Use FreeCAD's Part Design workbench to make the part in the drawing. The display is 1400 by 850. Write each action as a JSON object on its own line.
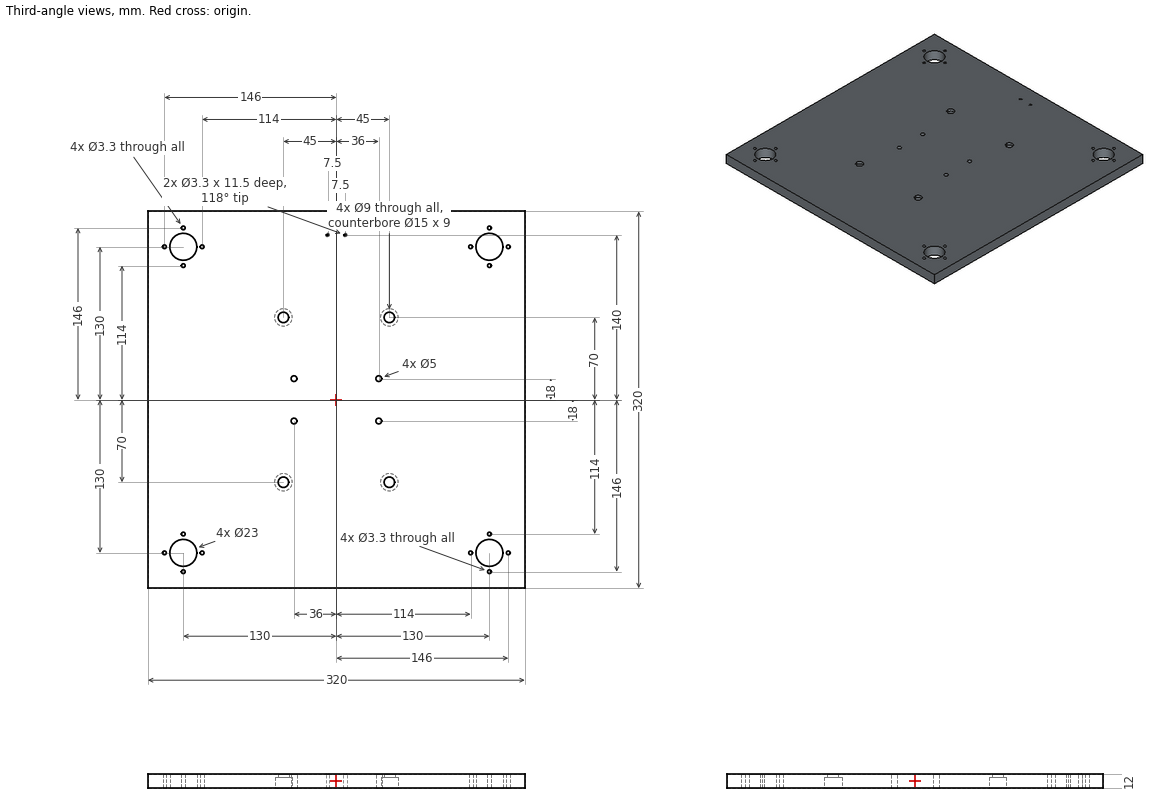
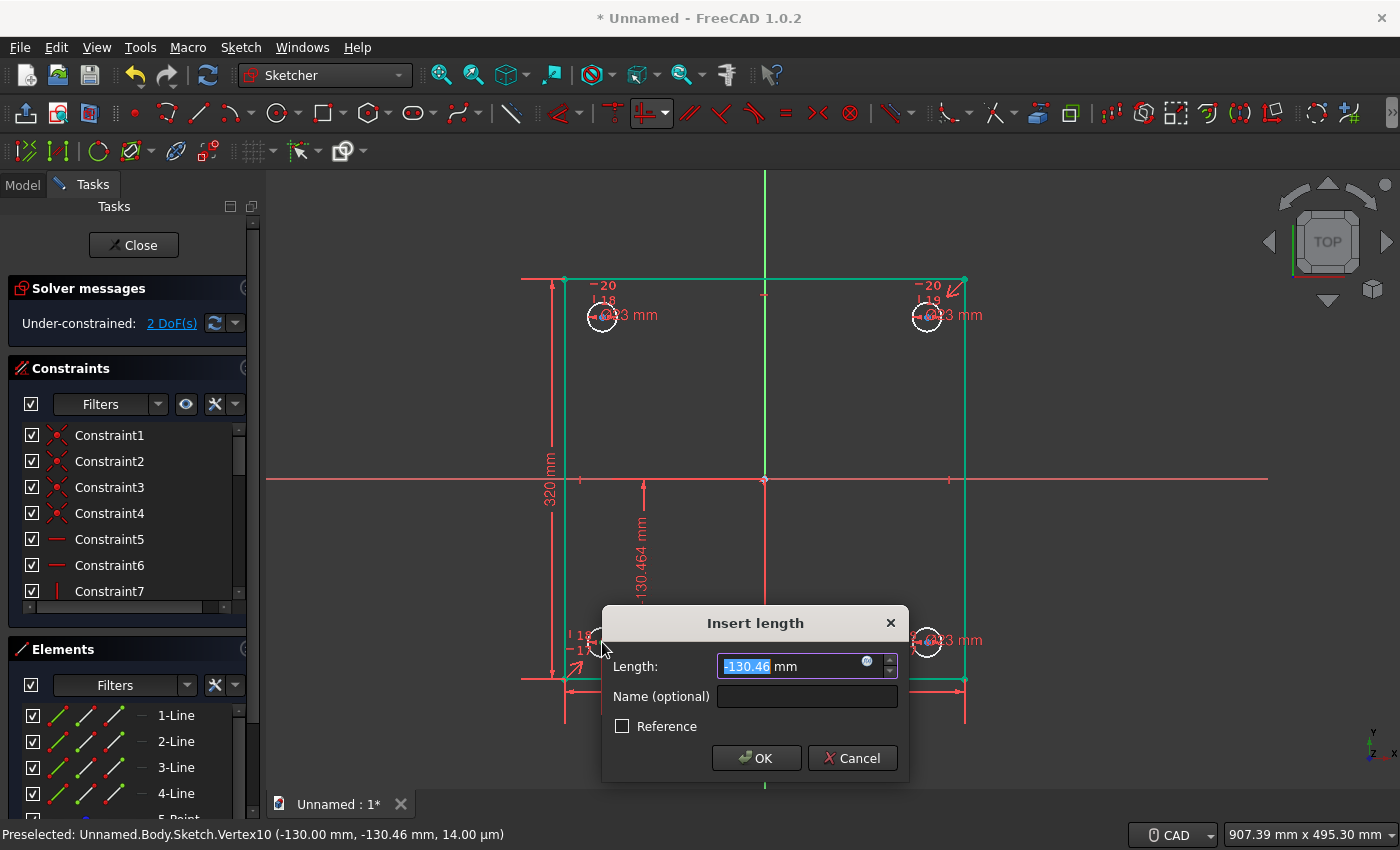
{"action": "type", "text": "-130"}
{"action": "key", "text": "Return"}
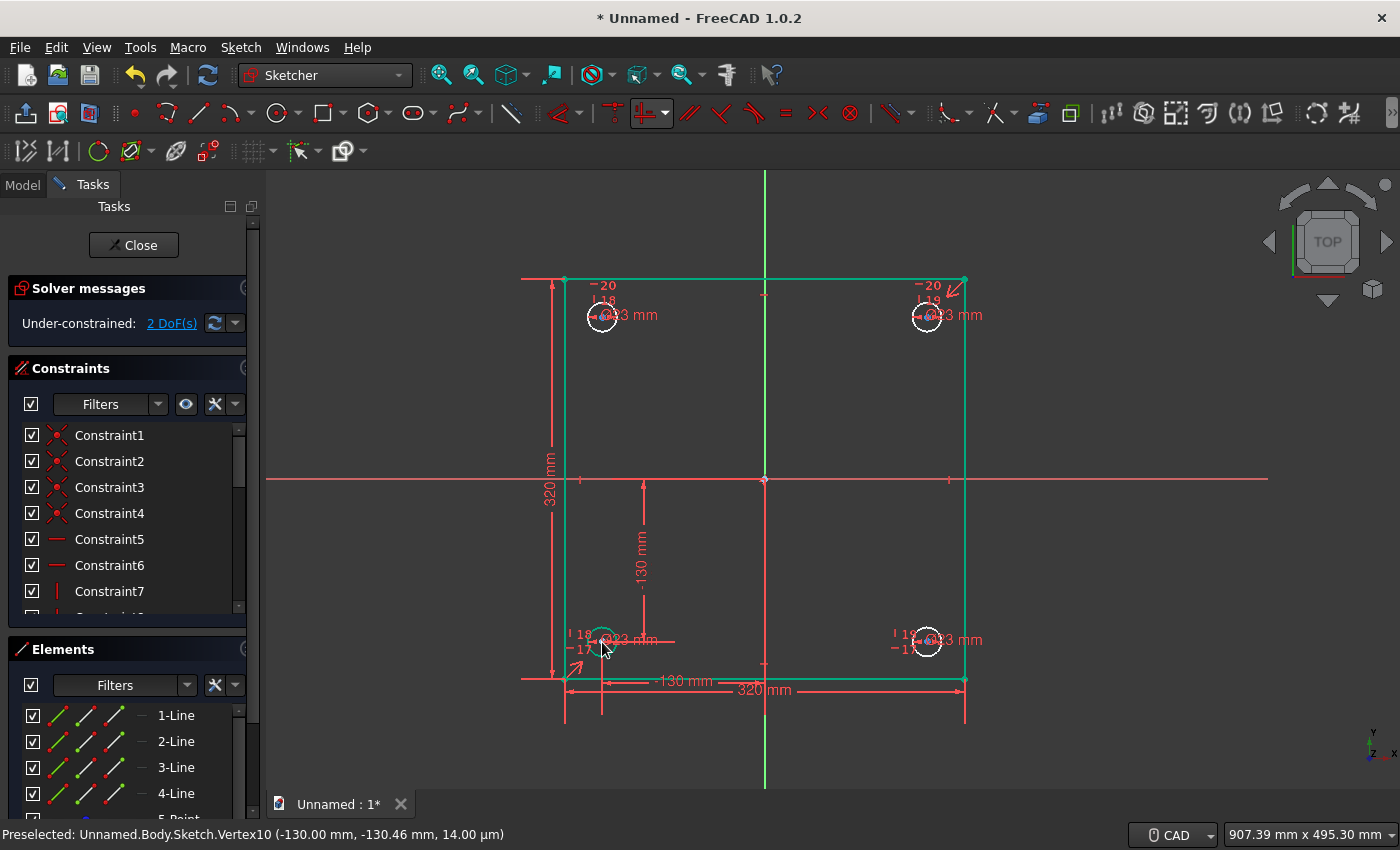
{"action": "left_click", "coordinate": [927, 642]}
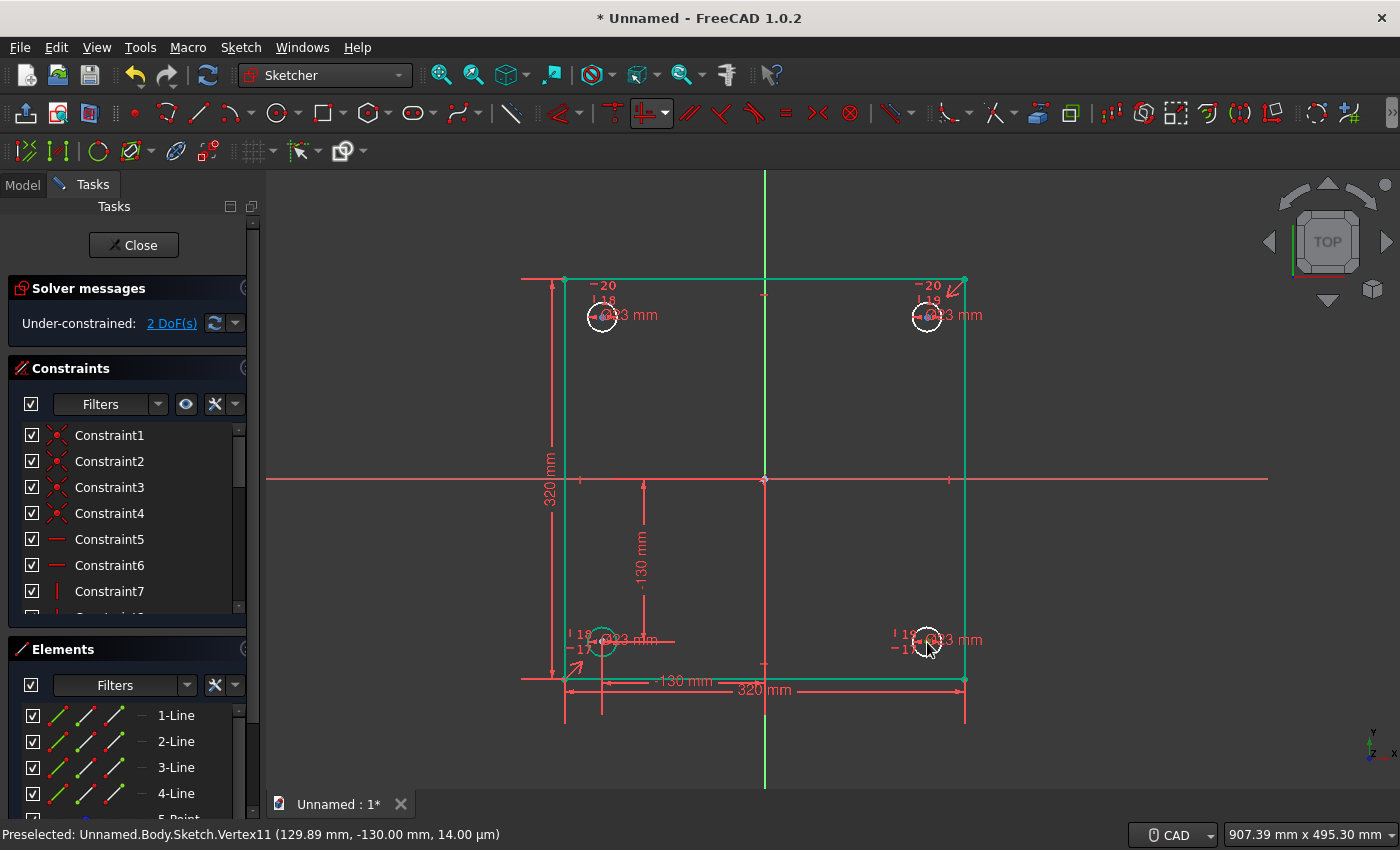
{"action": "left_click", "coordinate": [582, 114]}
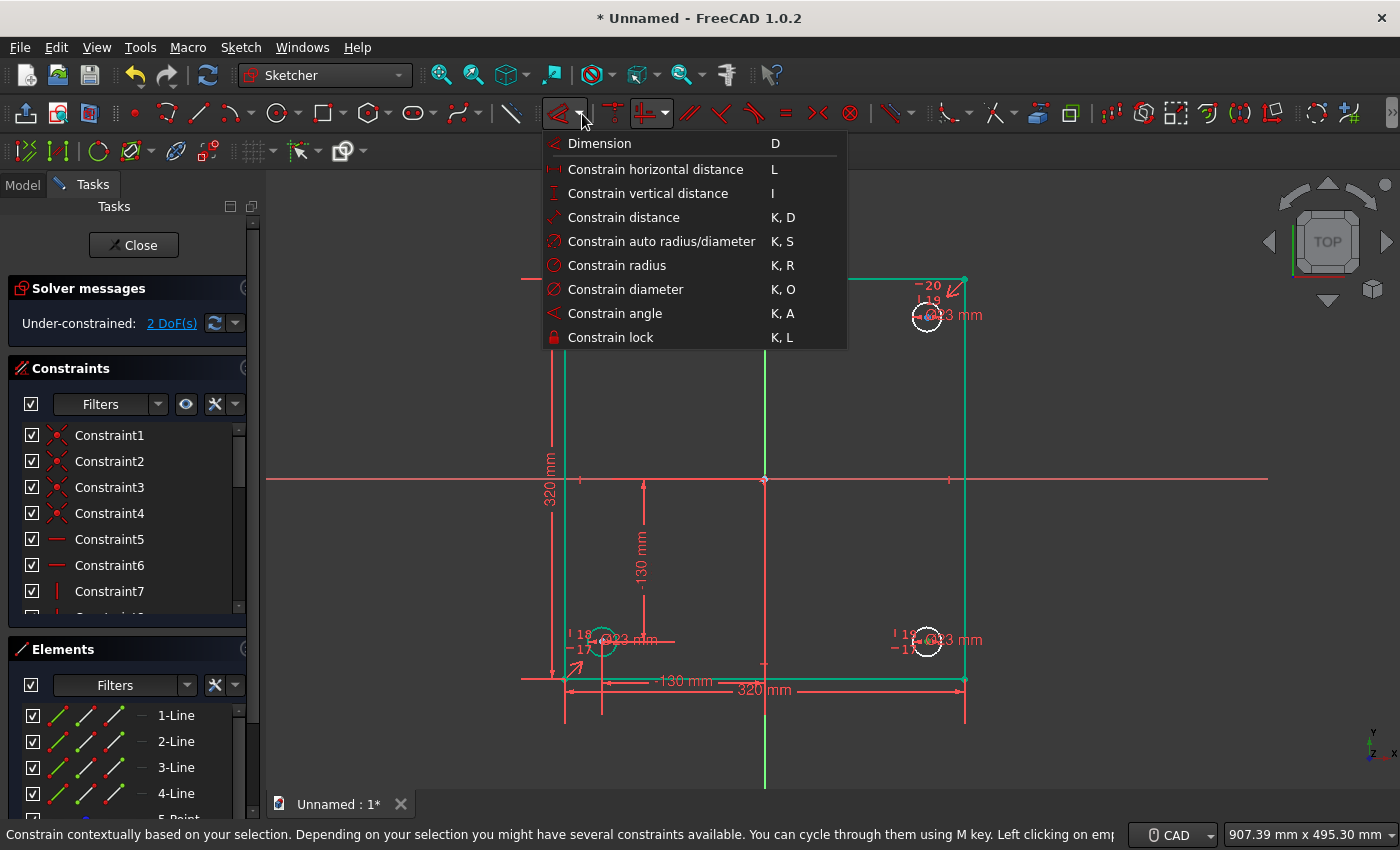
{"action": "left_click", "coordinate": [695, 169]}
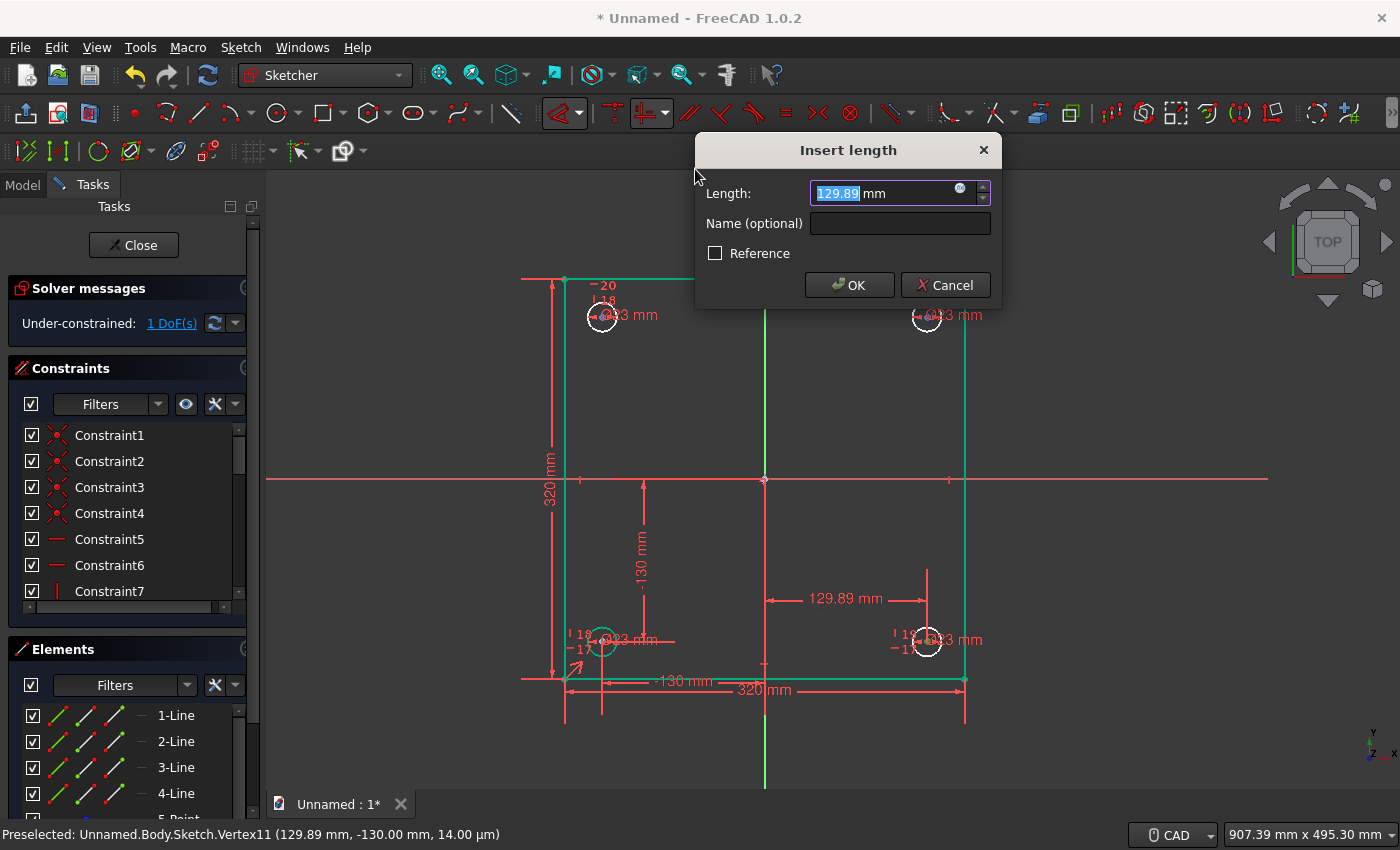
{"action": "type", "text": "130"}
{"action": "key", "text": "Return"}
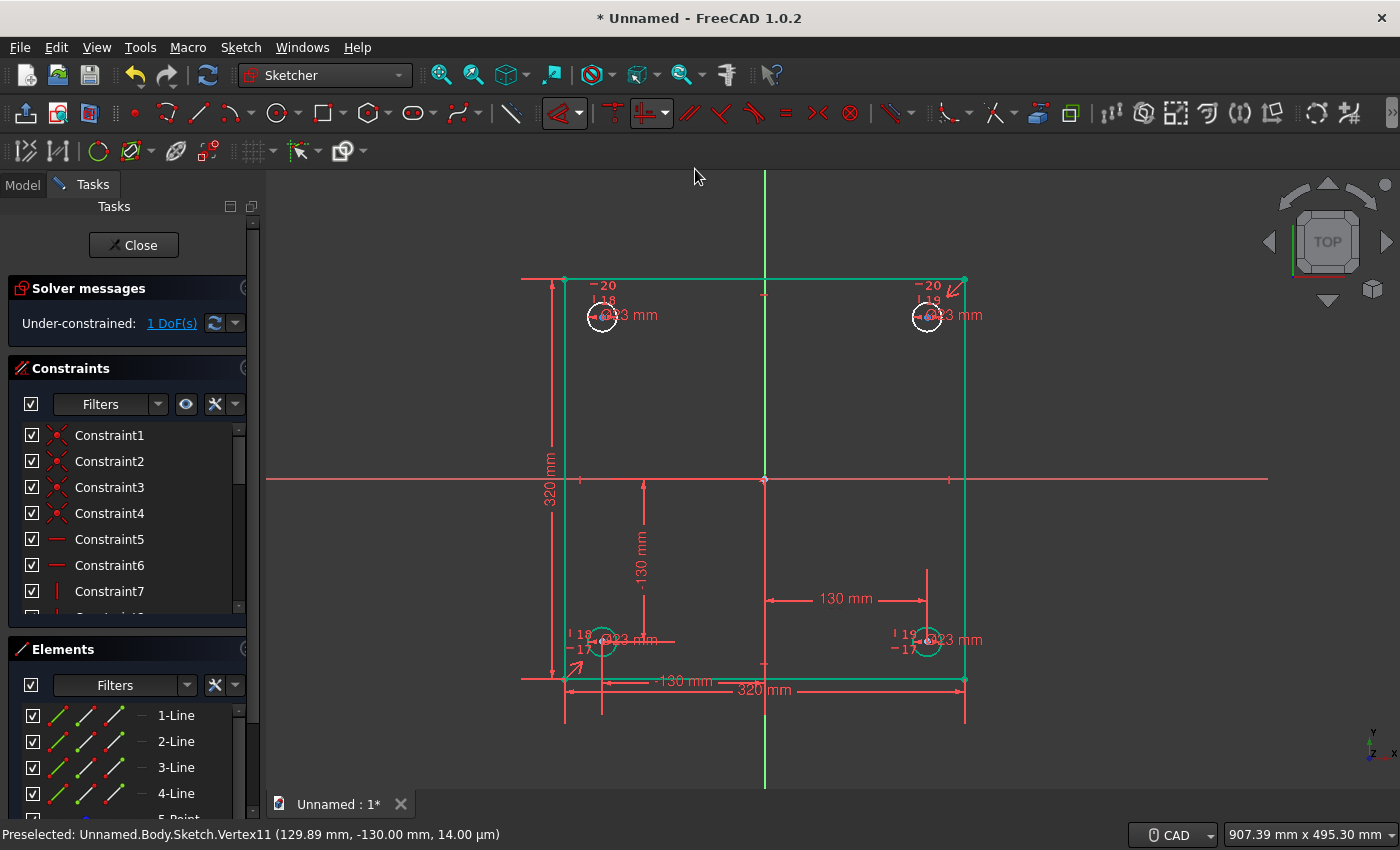
{"action": "left_click", "coordinate": [602, 317]}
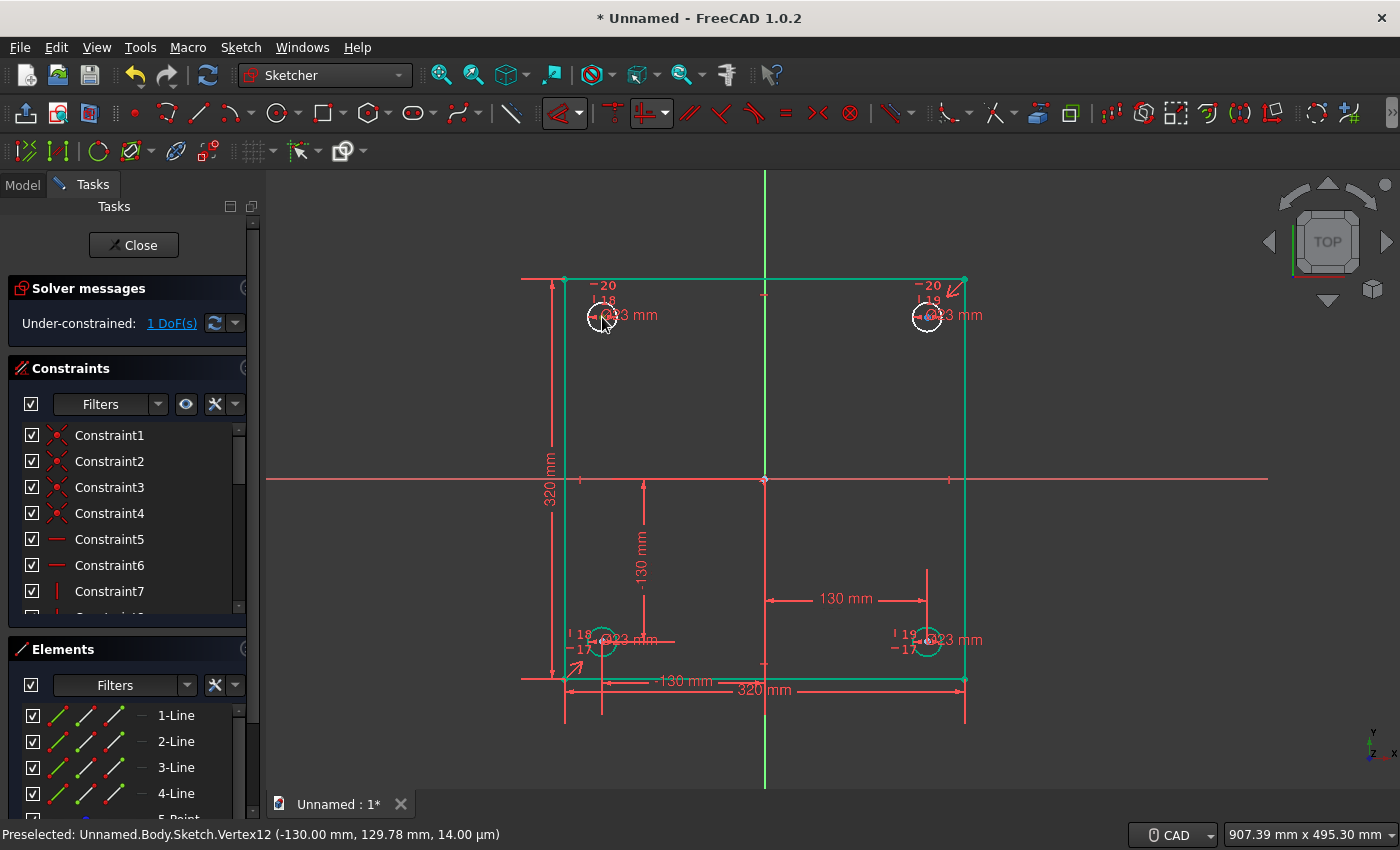
{"action": "key", "text": "i"}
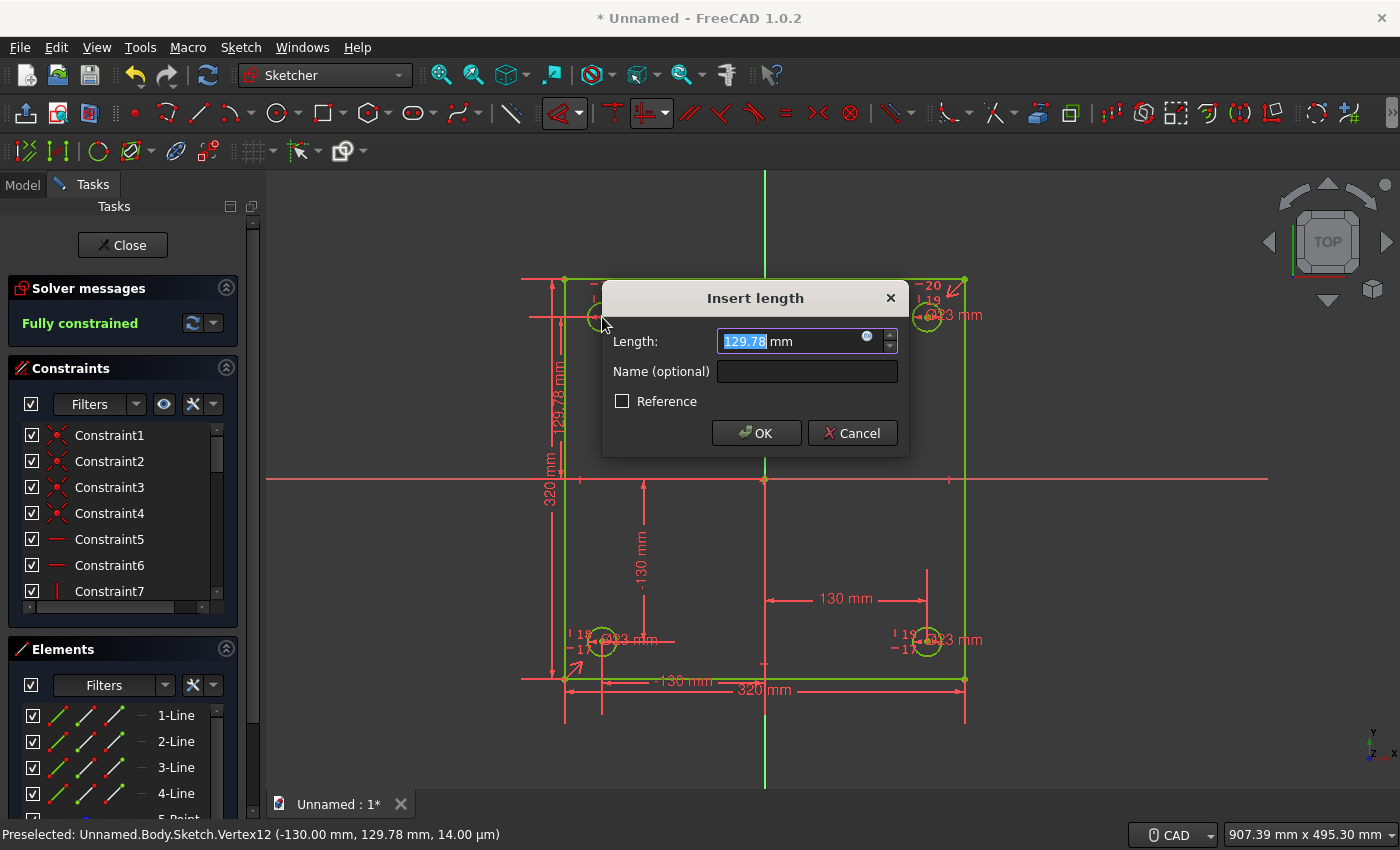
{"action": "type", "text": "130"}
{"action": "key", "text": "Return"}